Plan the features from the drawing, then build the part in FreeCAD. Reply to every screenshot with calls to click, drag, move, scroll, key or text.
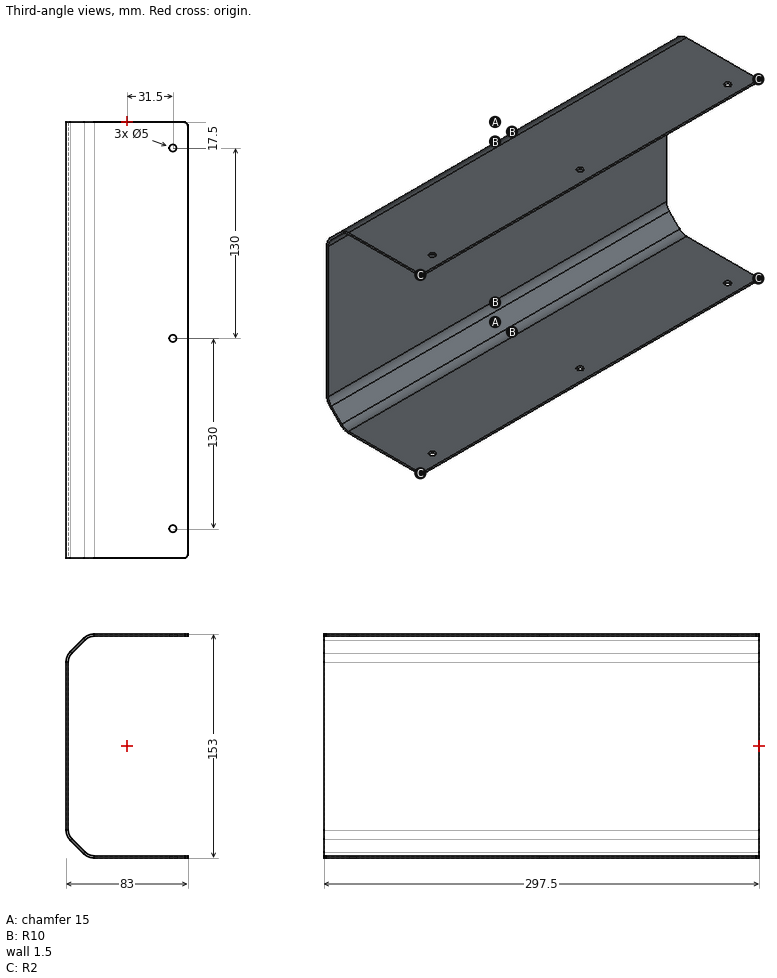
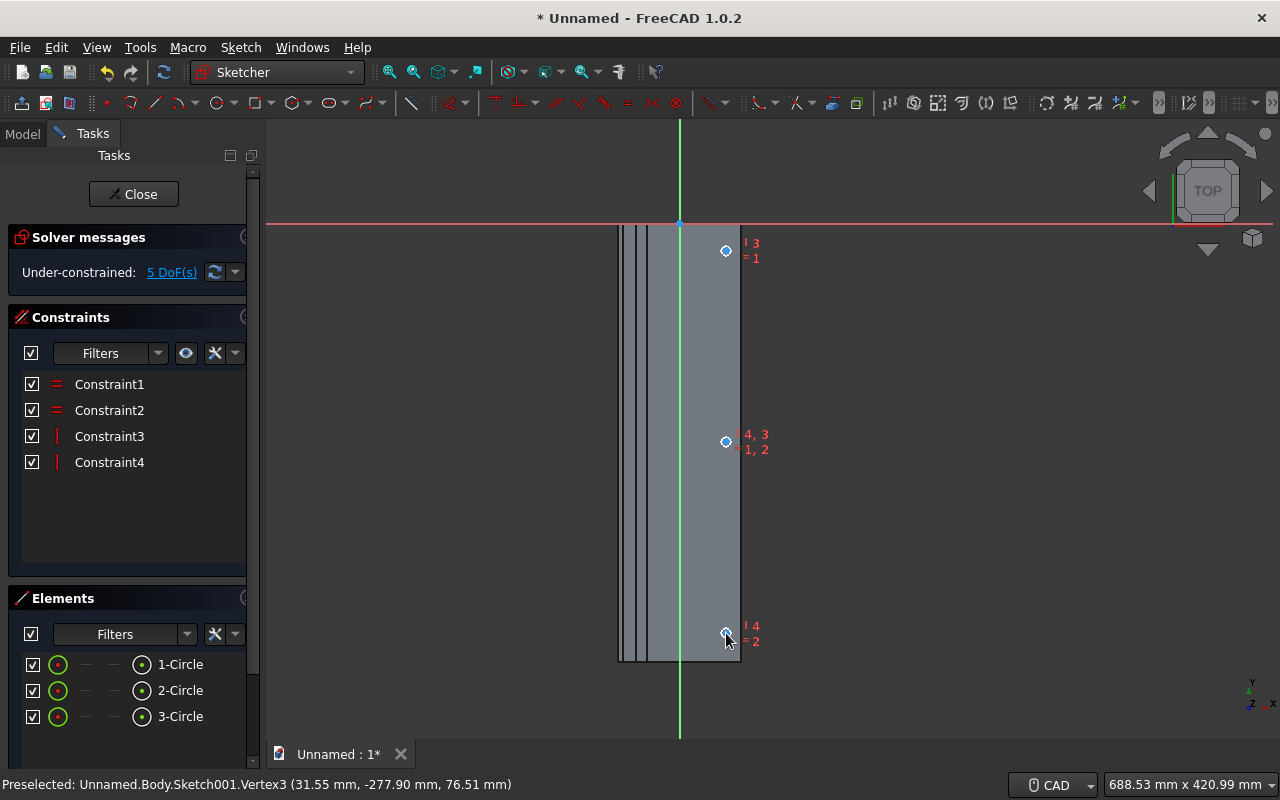
click(450, 104)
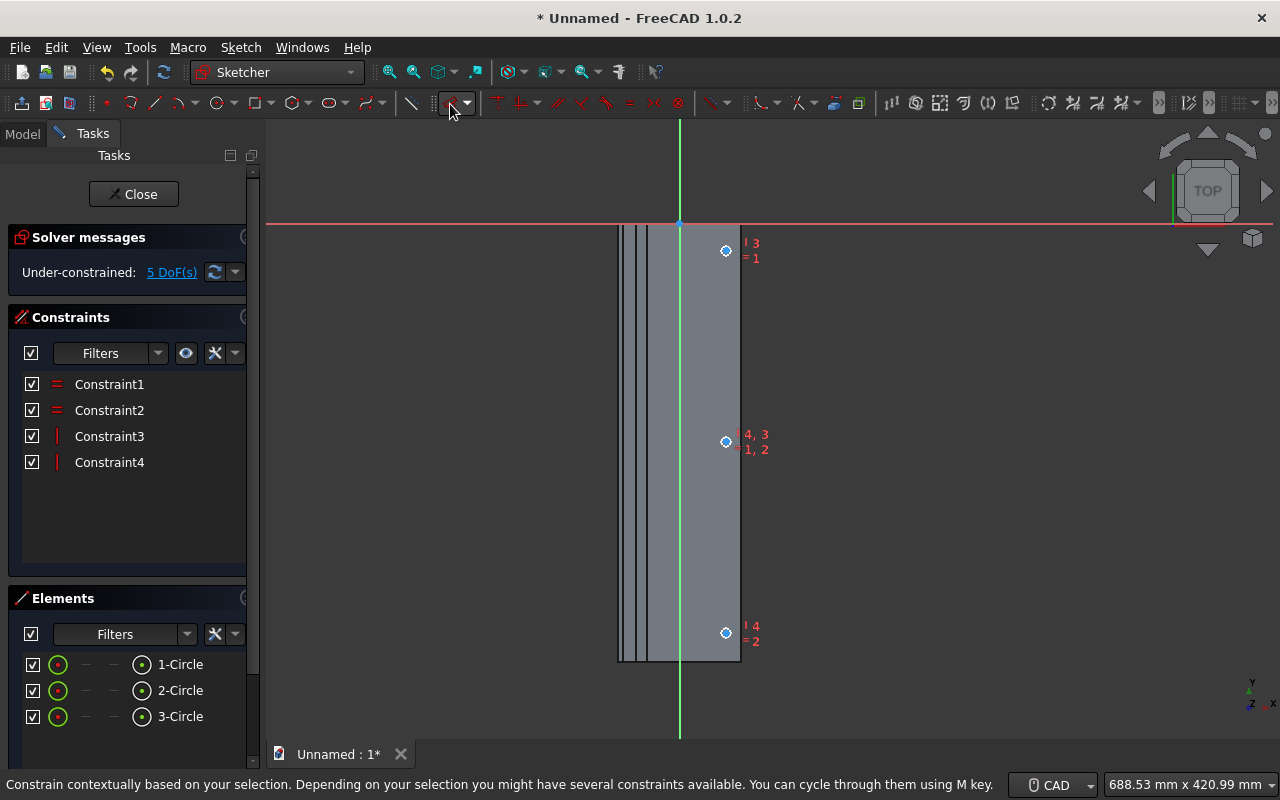
scroll(726, 256, up, 9)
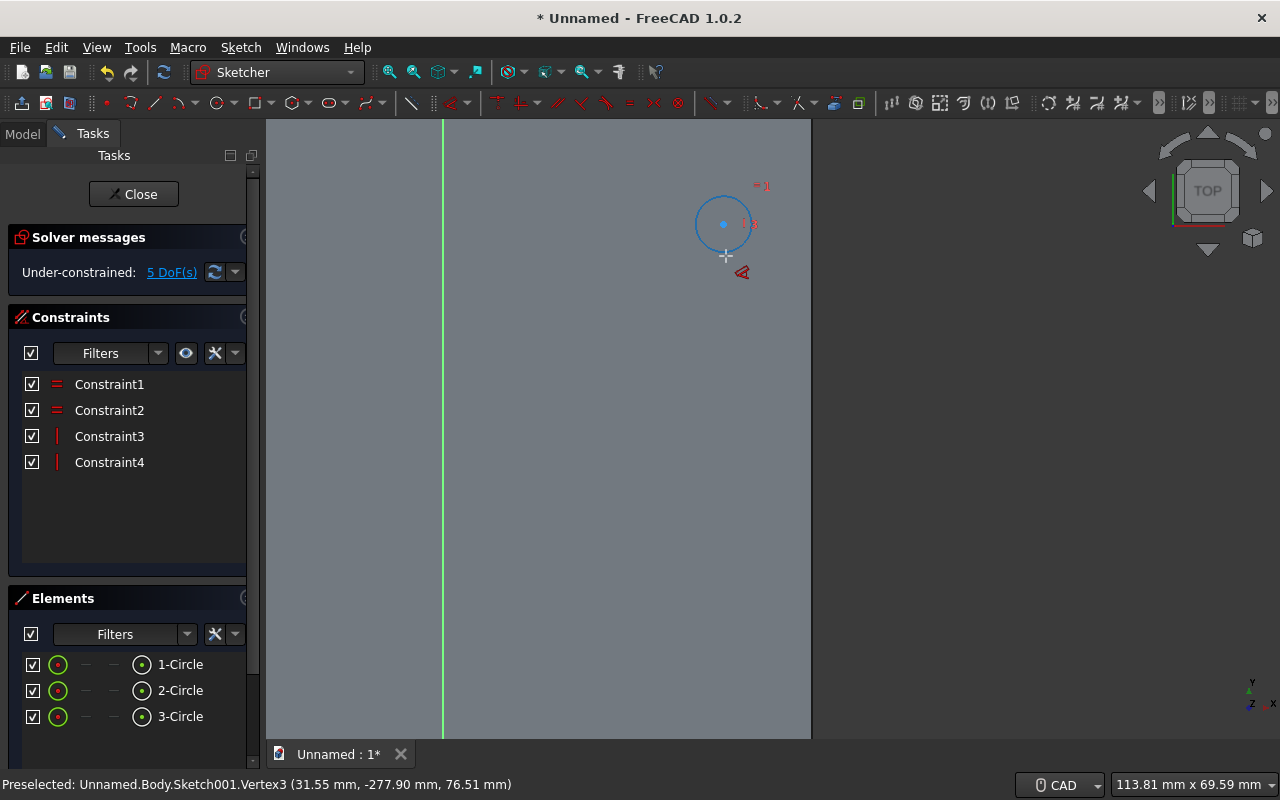
click(723, 252)
click(722, 284)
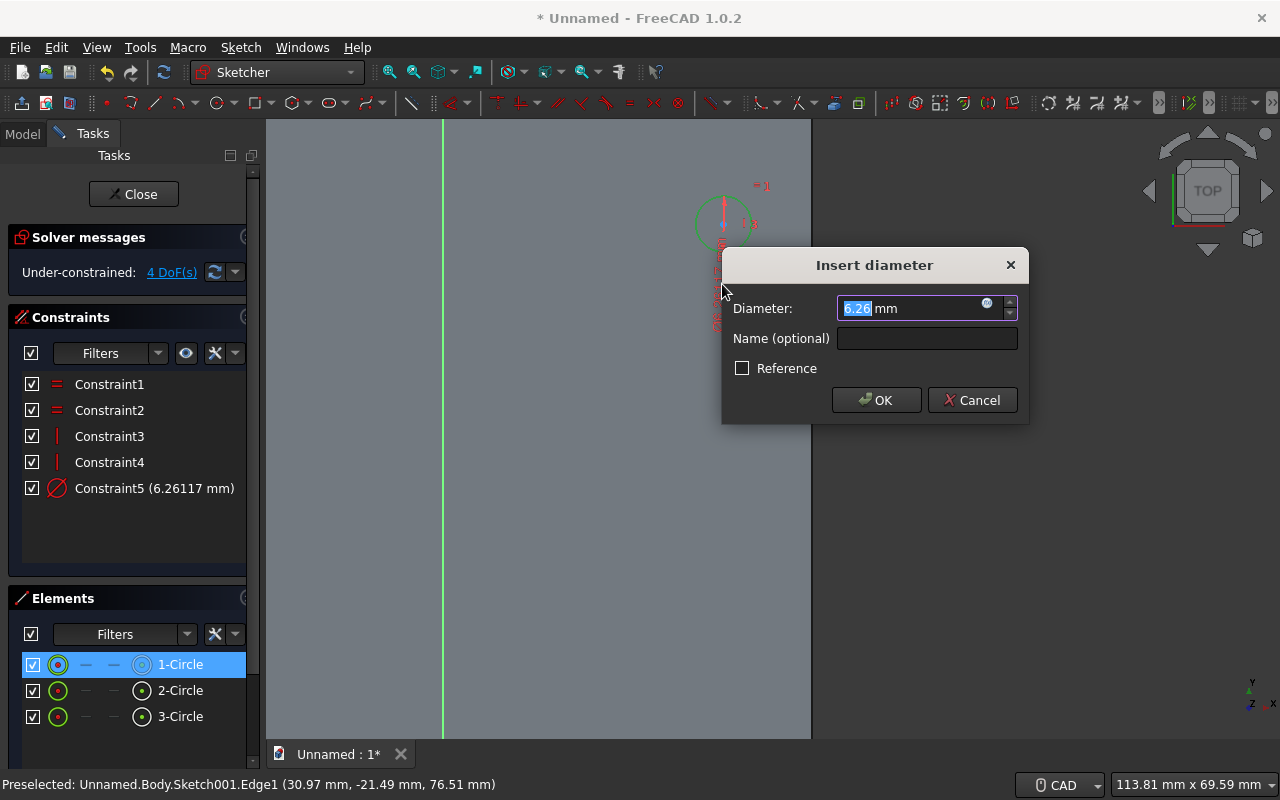
text(5)
key(Return)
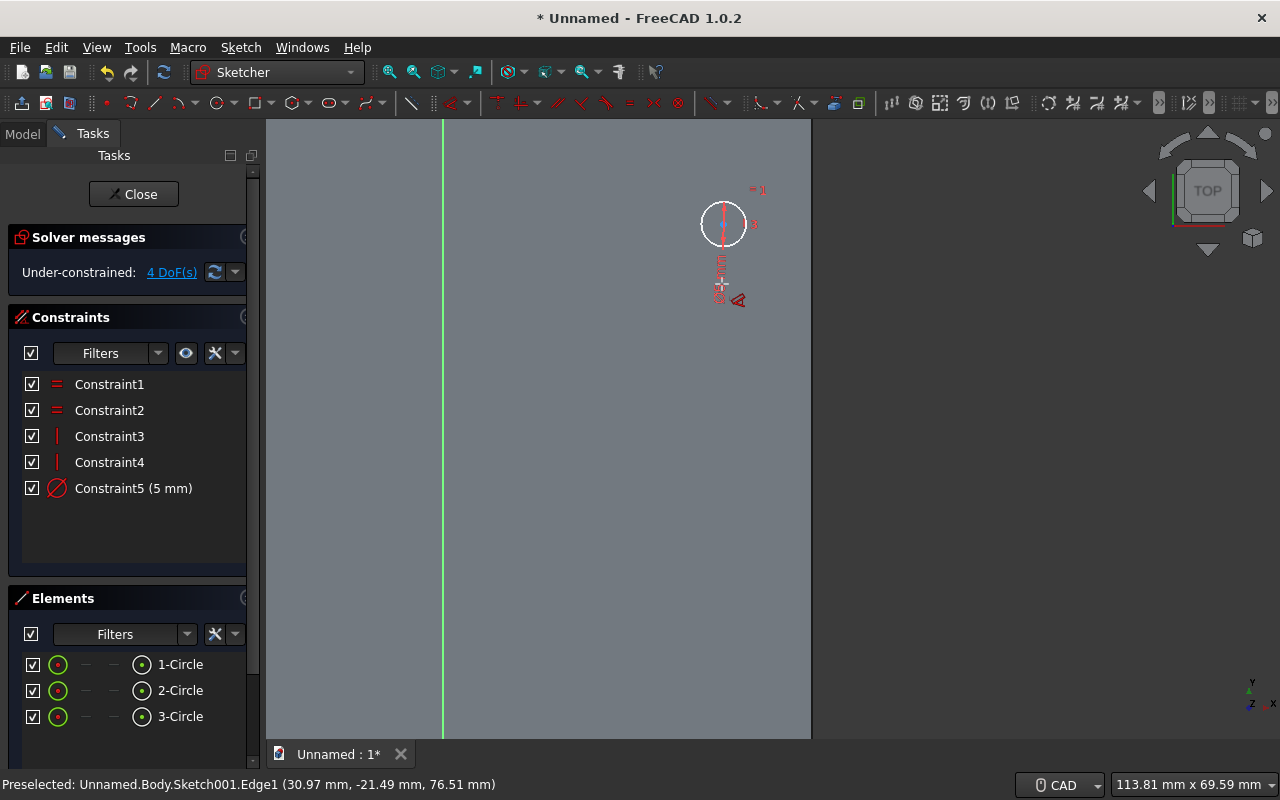
scroll(726, 255, down, 9)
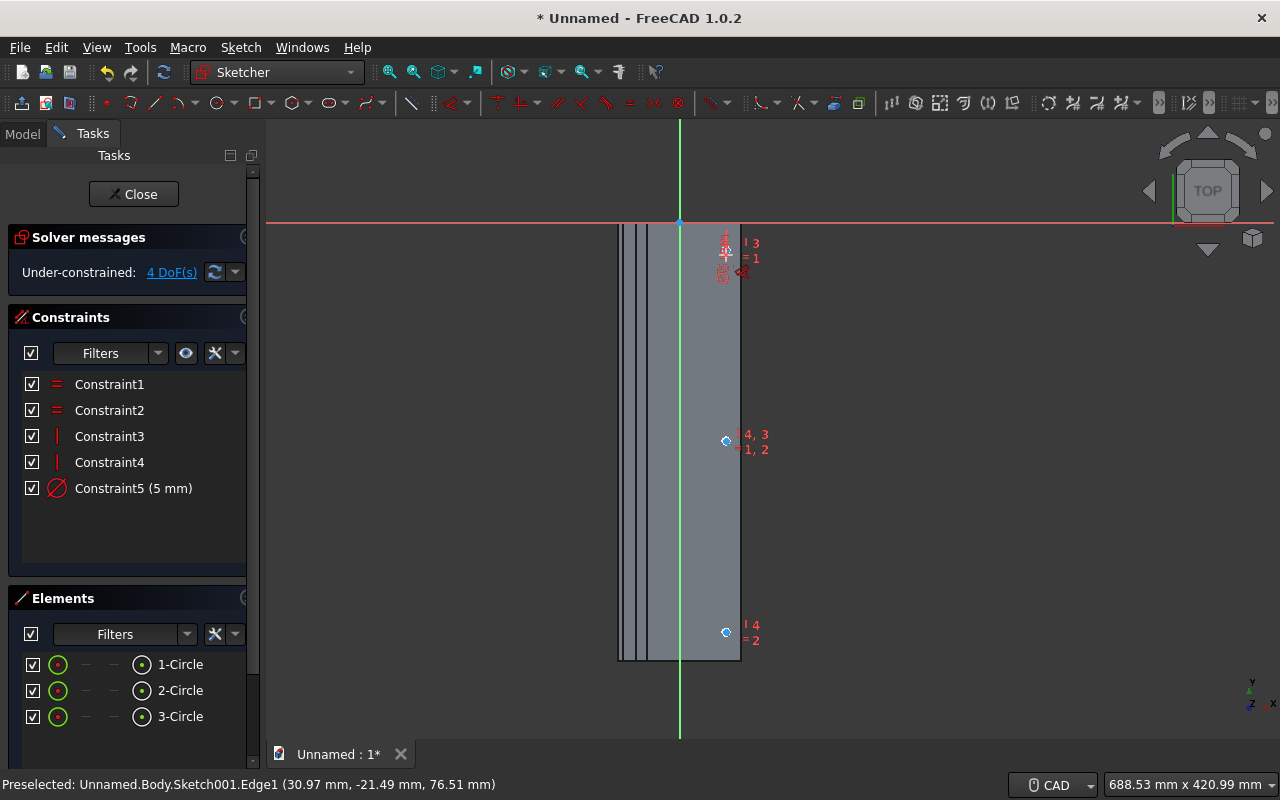
click(726, 250)
click(703, 189)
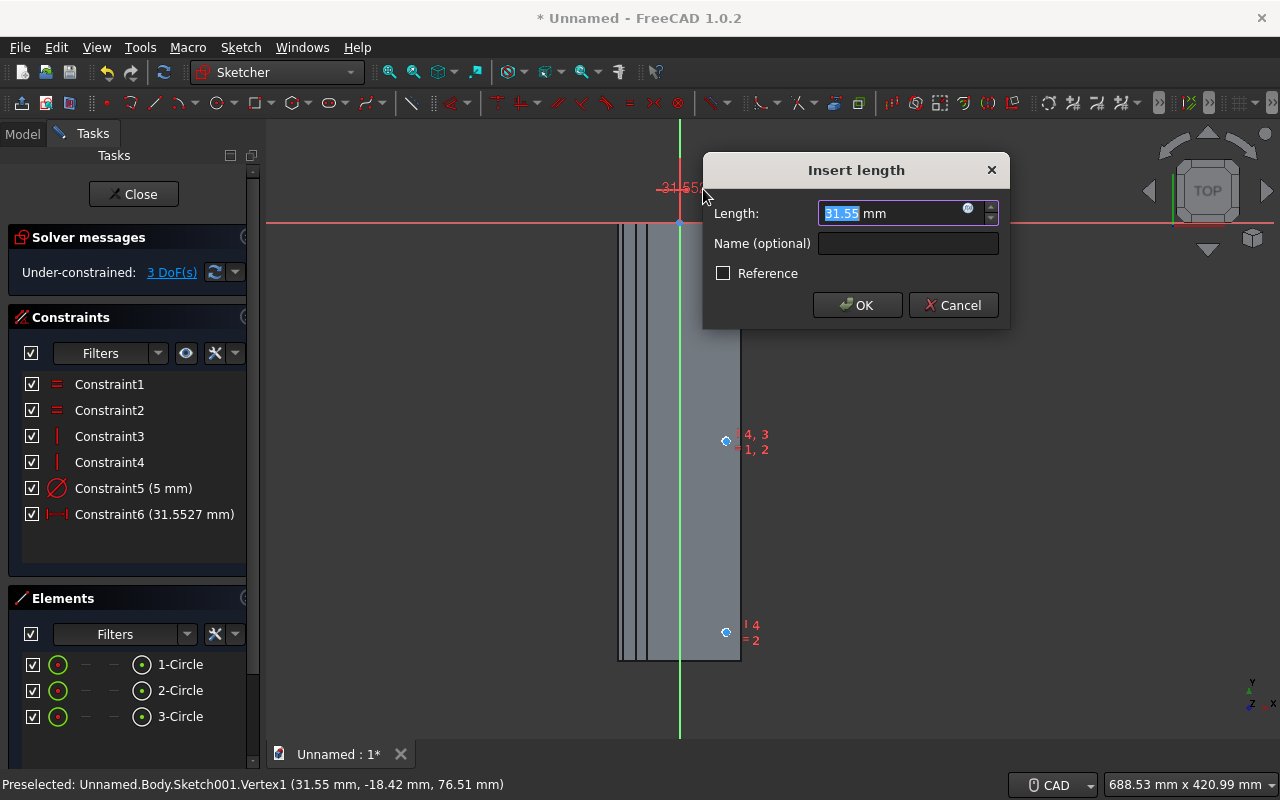
text(31.5)
key(Return)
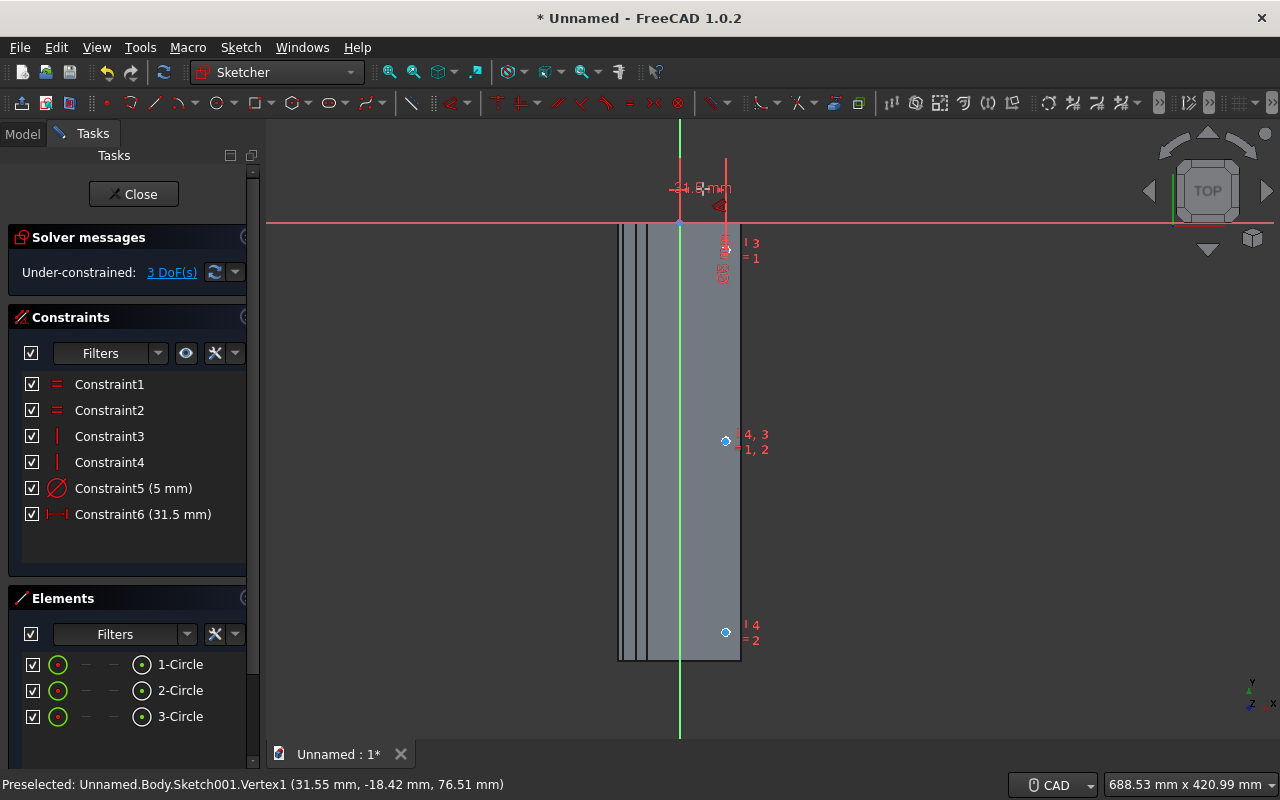
scroll(726, 250, up, 3)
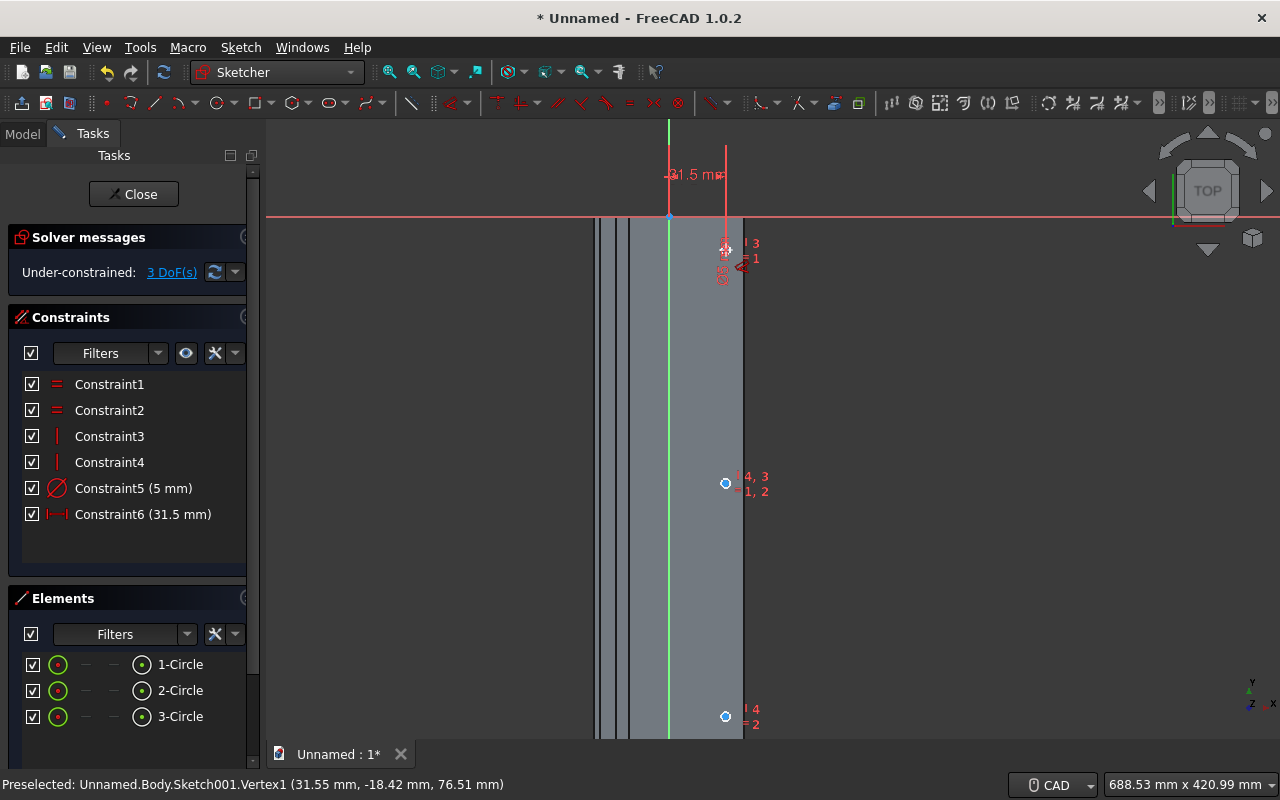
click(725, 250)
click(607, 225)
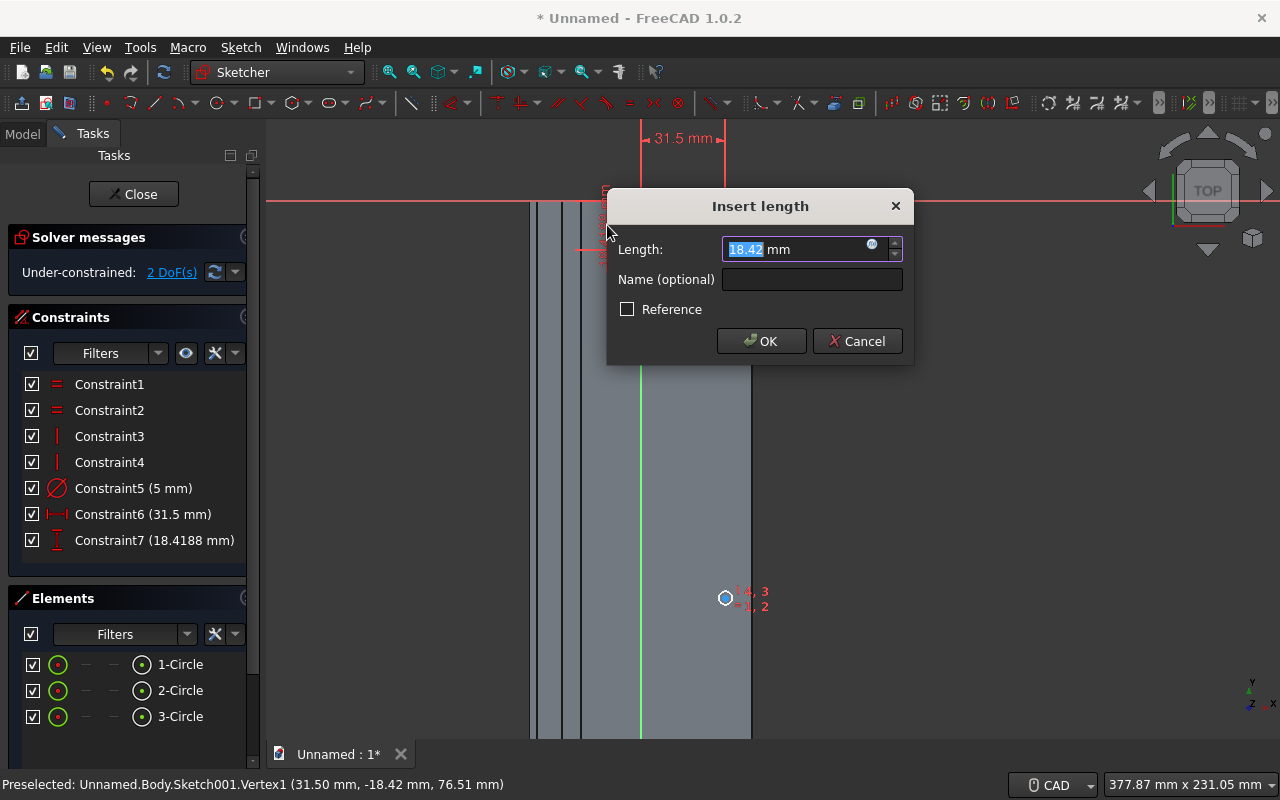
text(17.5)
key(Return)